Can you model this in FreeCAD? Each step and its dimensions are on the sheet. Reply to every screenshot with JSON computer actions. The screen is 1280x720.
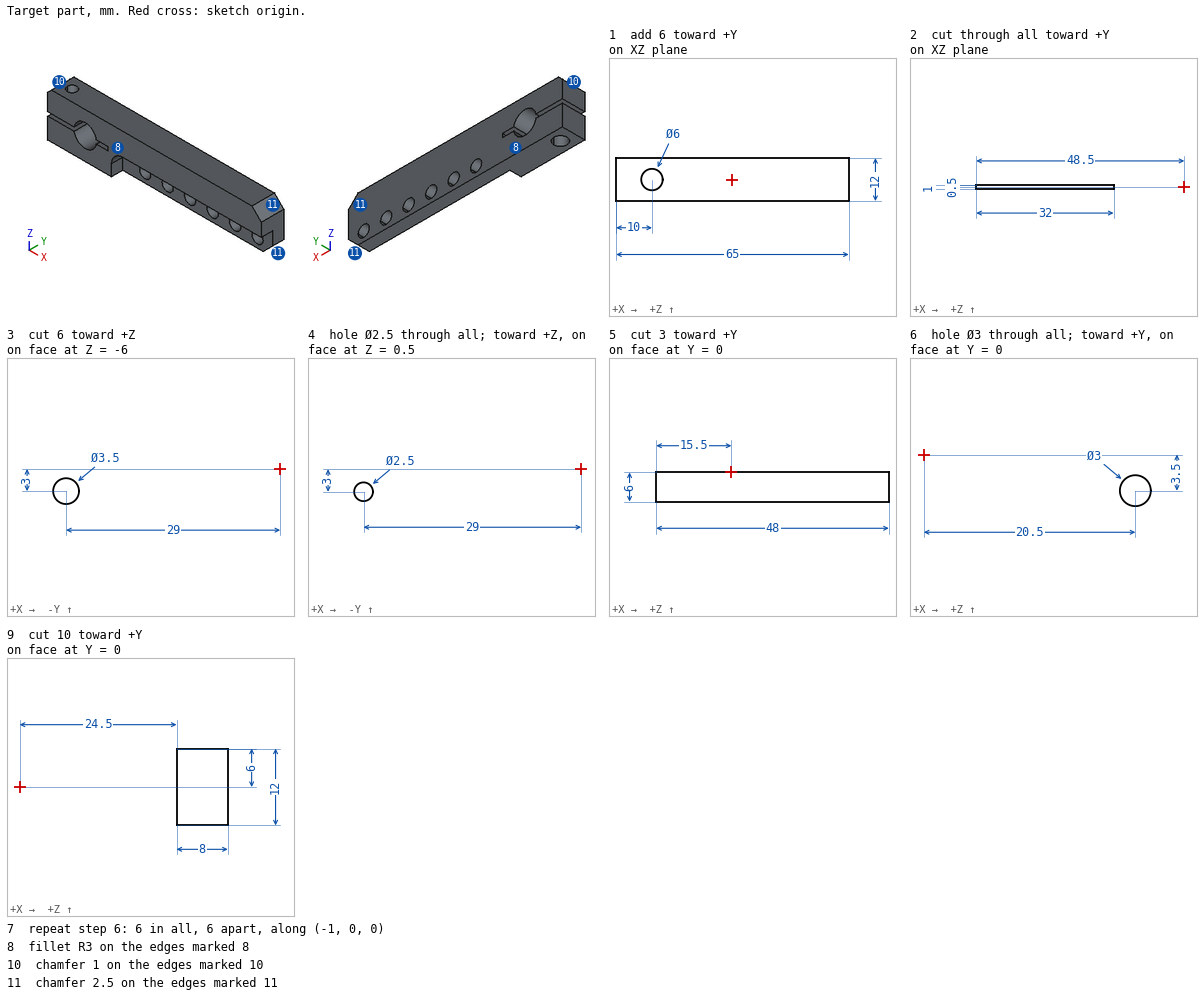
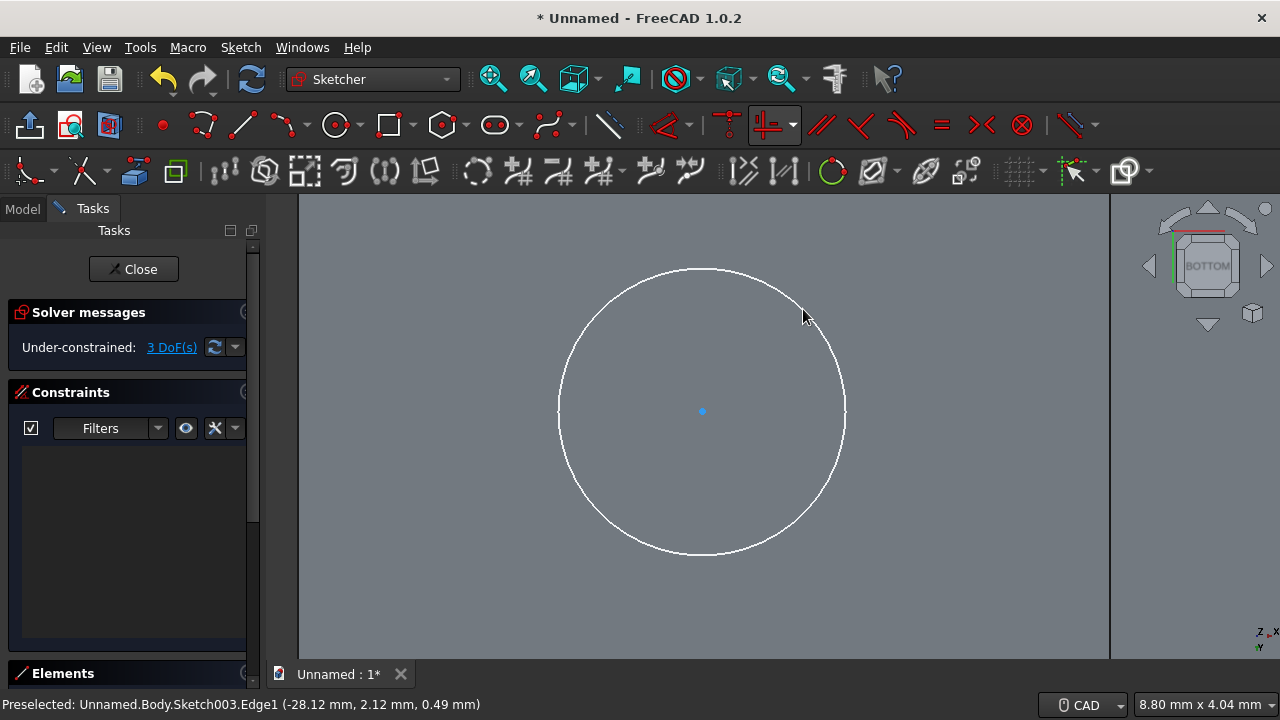
{"action": "left_click", "coordinate": [664, 126]}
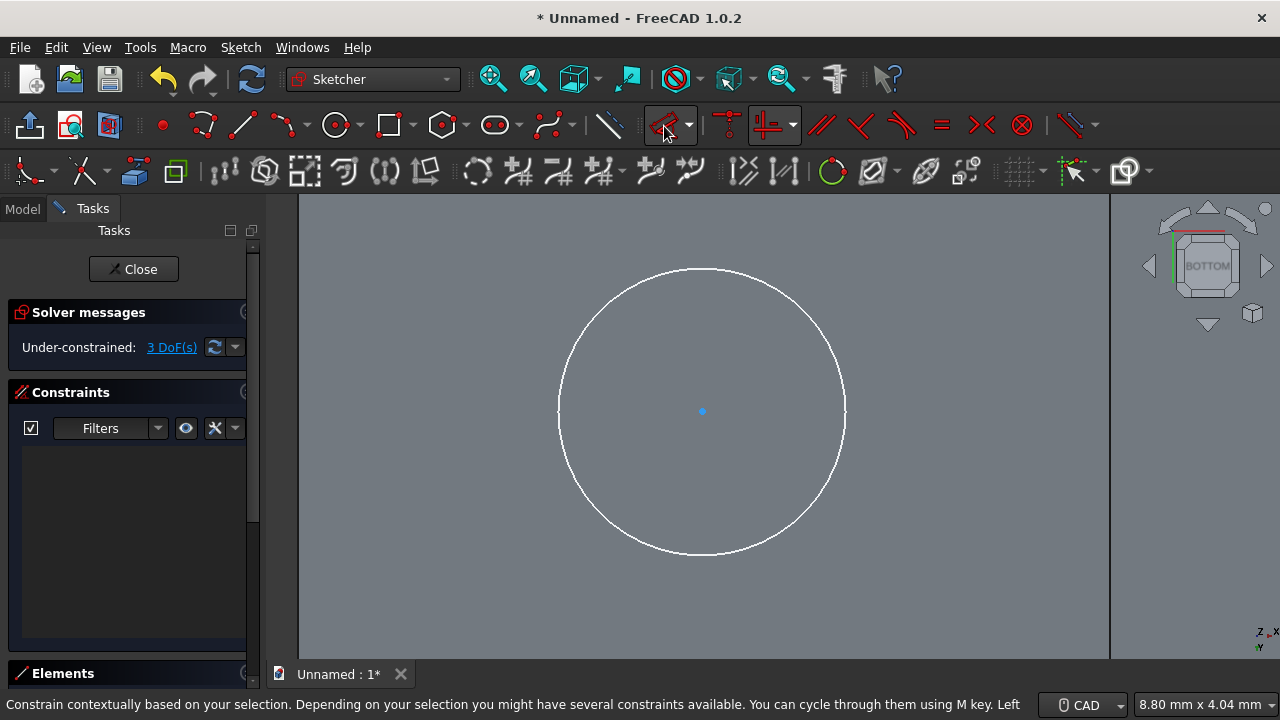
{"action": "left_click", "coordinate": [803, 310]}
{"action": "left_click", "coordinate": [826, 287]}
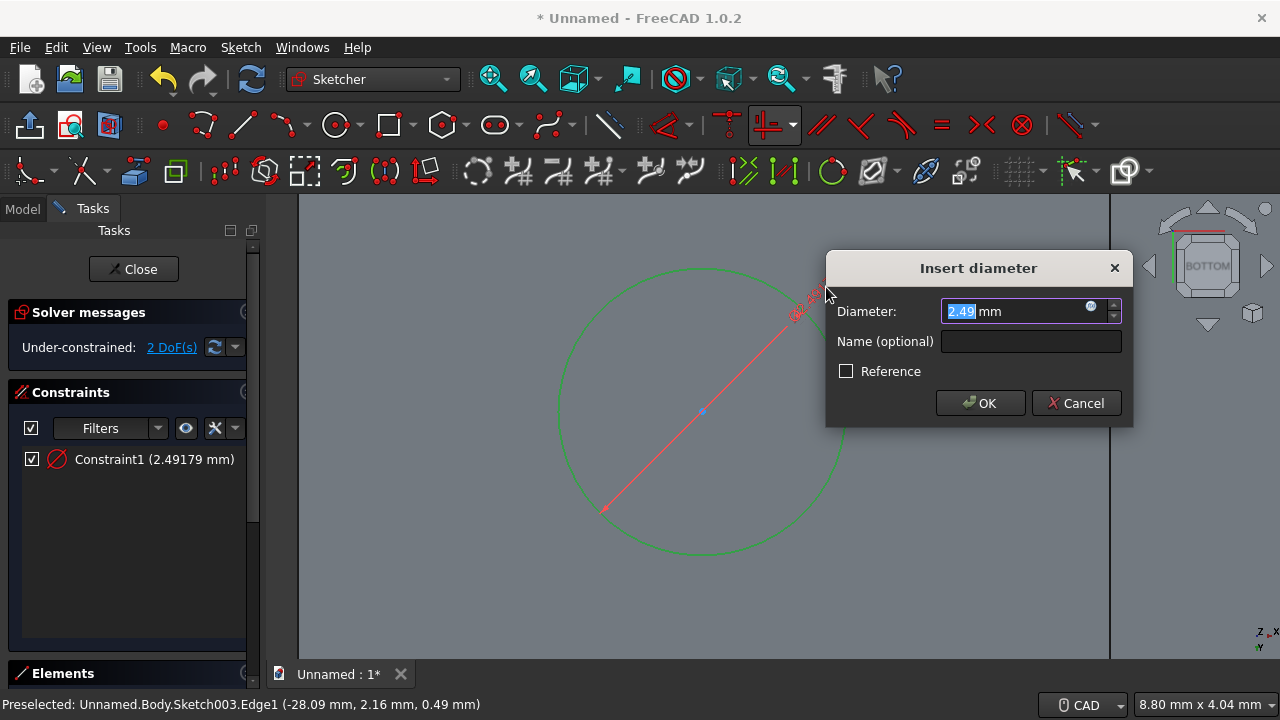
{"action": "type", "text": "2.5"}
{"action": "key", "text": "Return"}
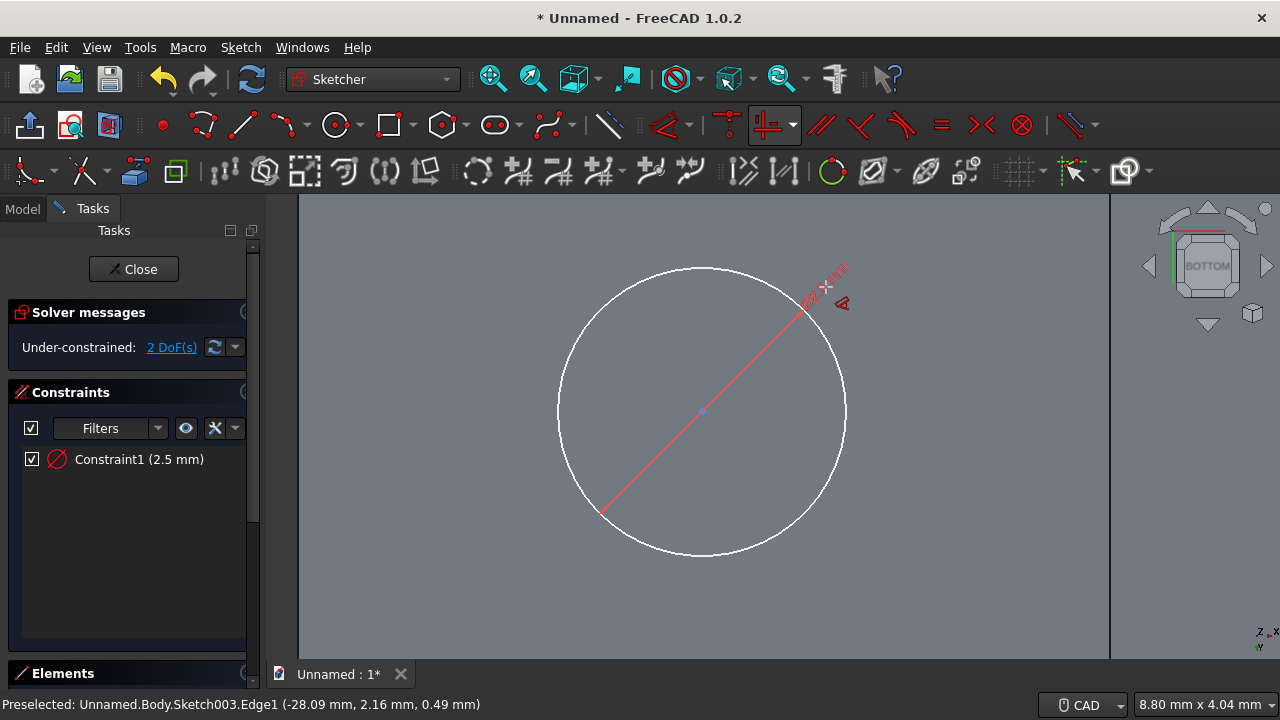
{"action": "left_click", "coordinate": [702, 412]}
{"action": "left_click", "coordinate": [668, 317]}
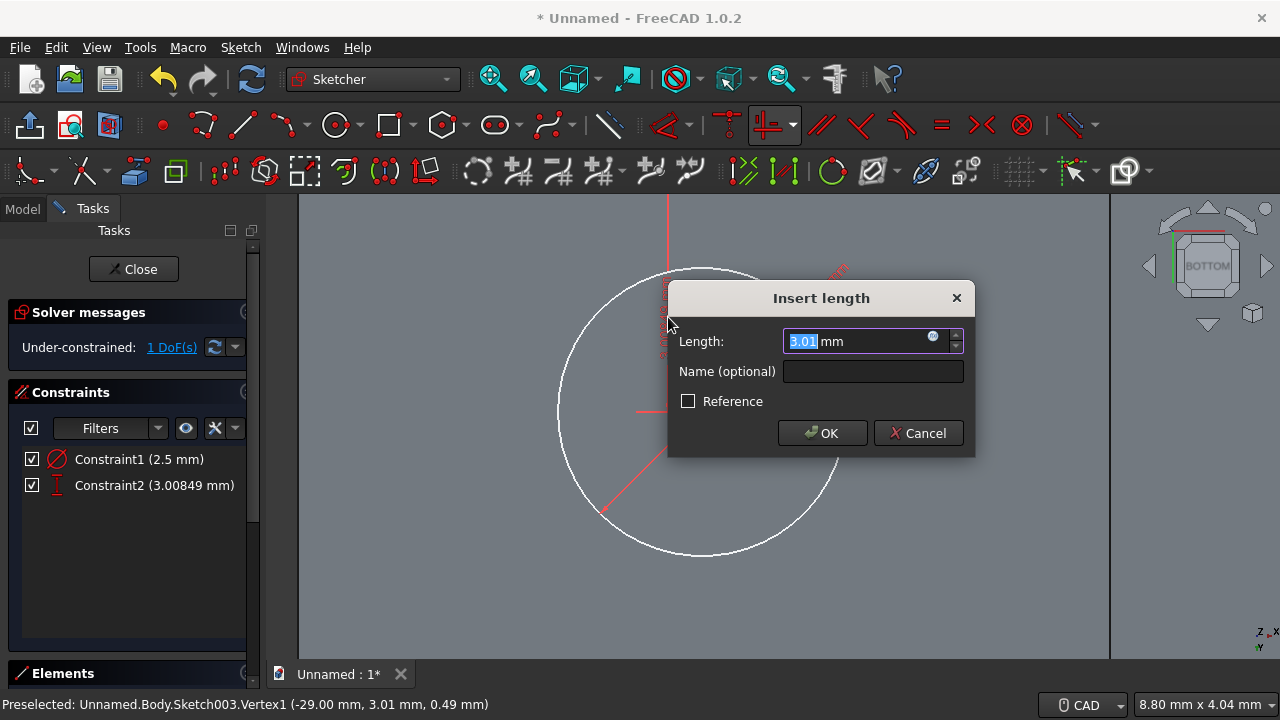
{"action": "type", "text": "3"}
{"action": "key", "text": "Return"}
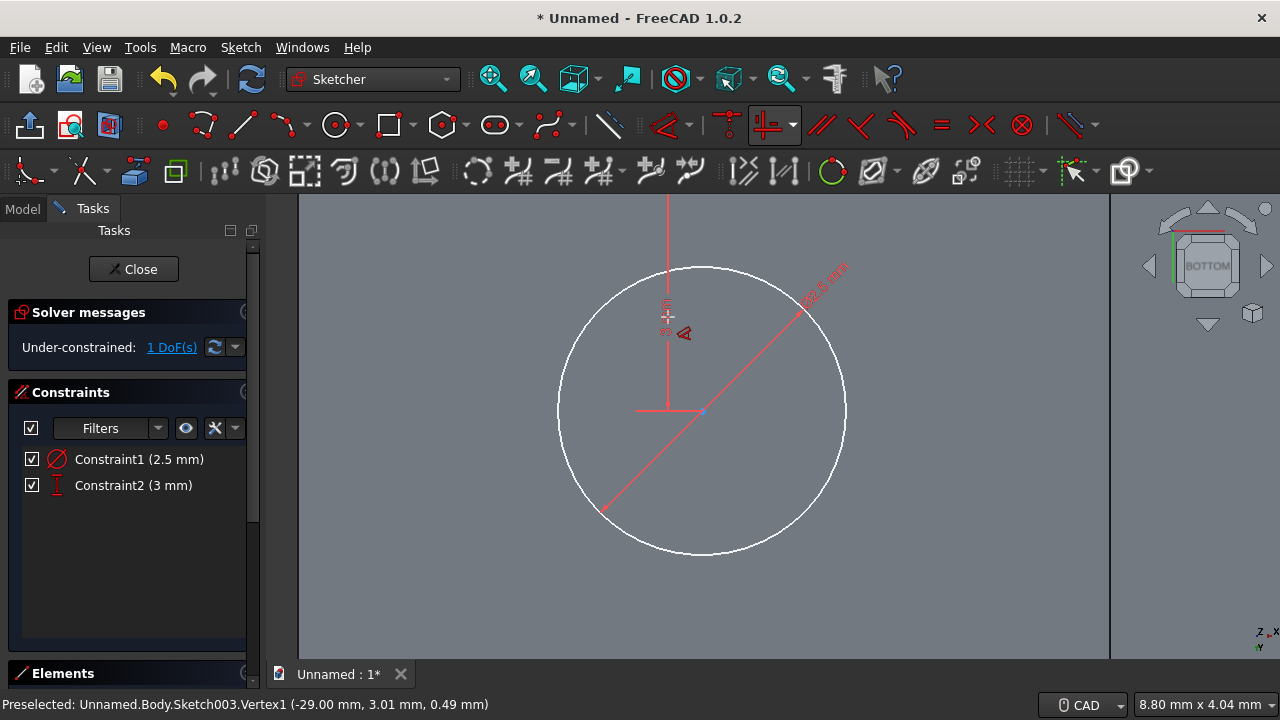
{"action": "left_click", "coordinate": [702, 411]}
{"action": "left_click", "coordinate": [909, 445]}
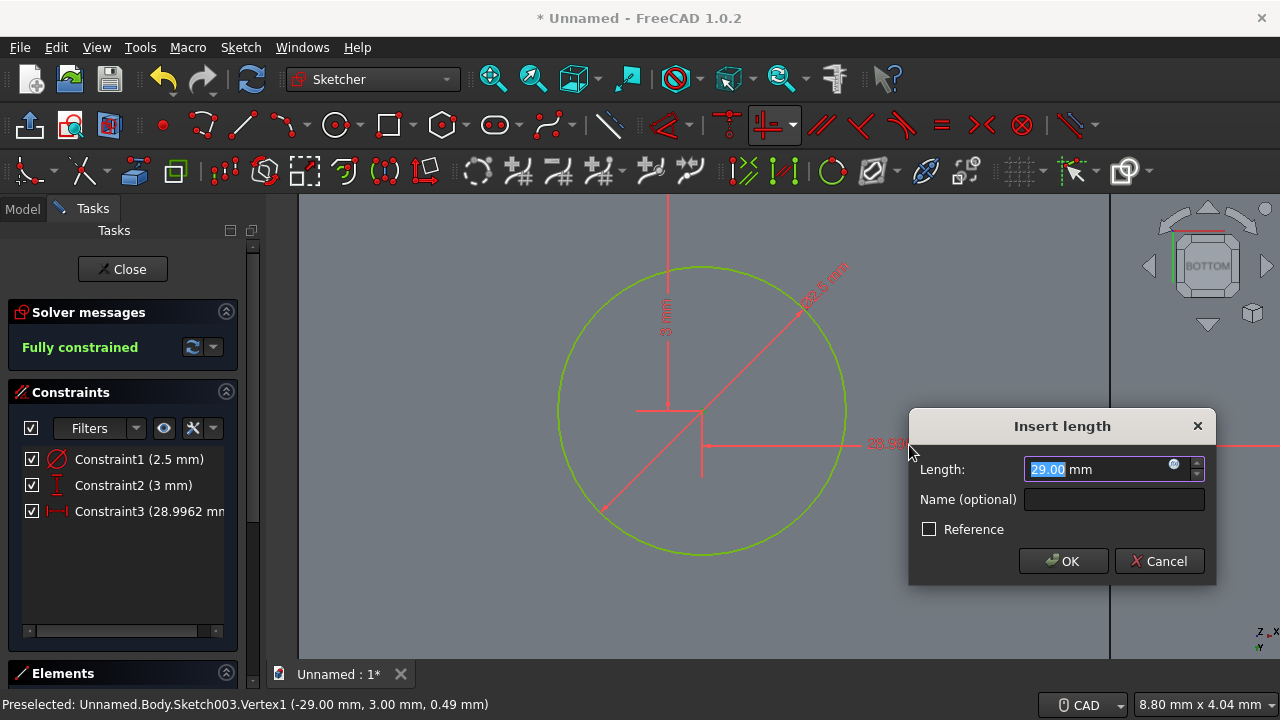
{"action": "type", "text": "29"}
{"action": "key", "text": "Return"}
{"action": "key", "text": "Escape"}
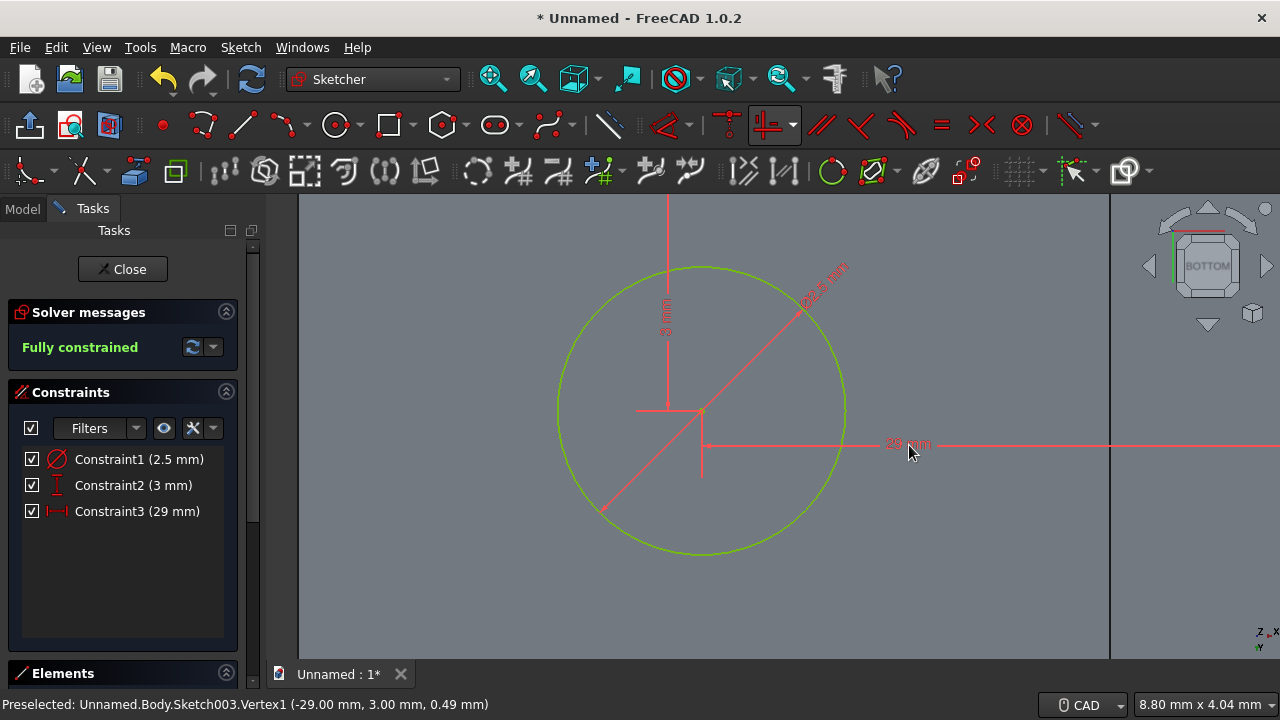
{"action": "left_click", "coordinate": [123, 269]}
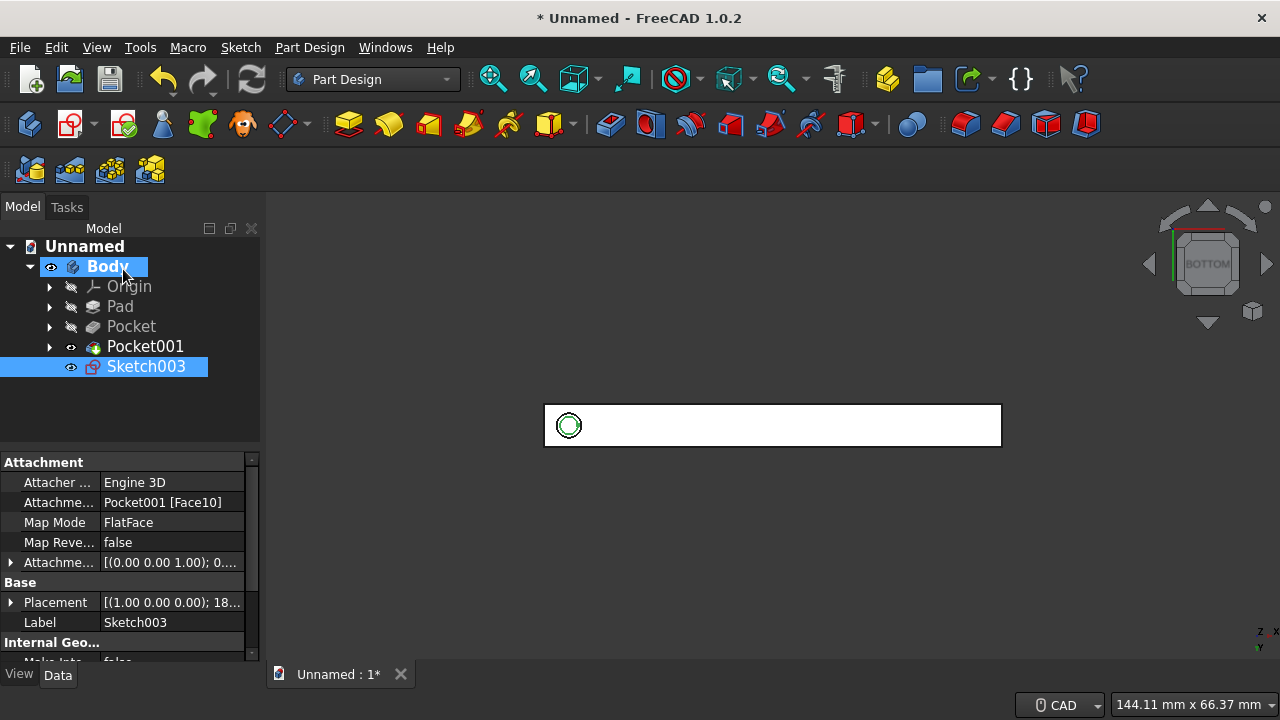
{"action": "left_click", "coordinate": [652, 124]}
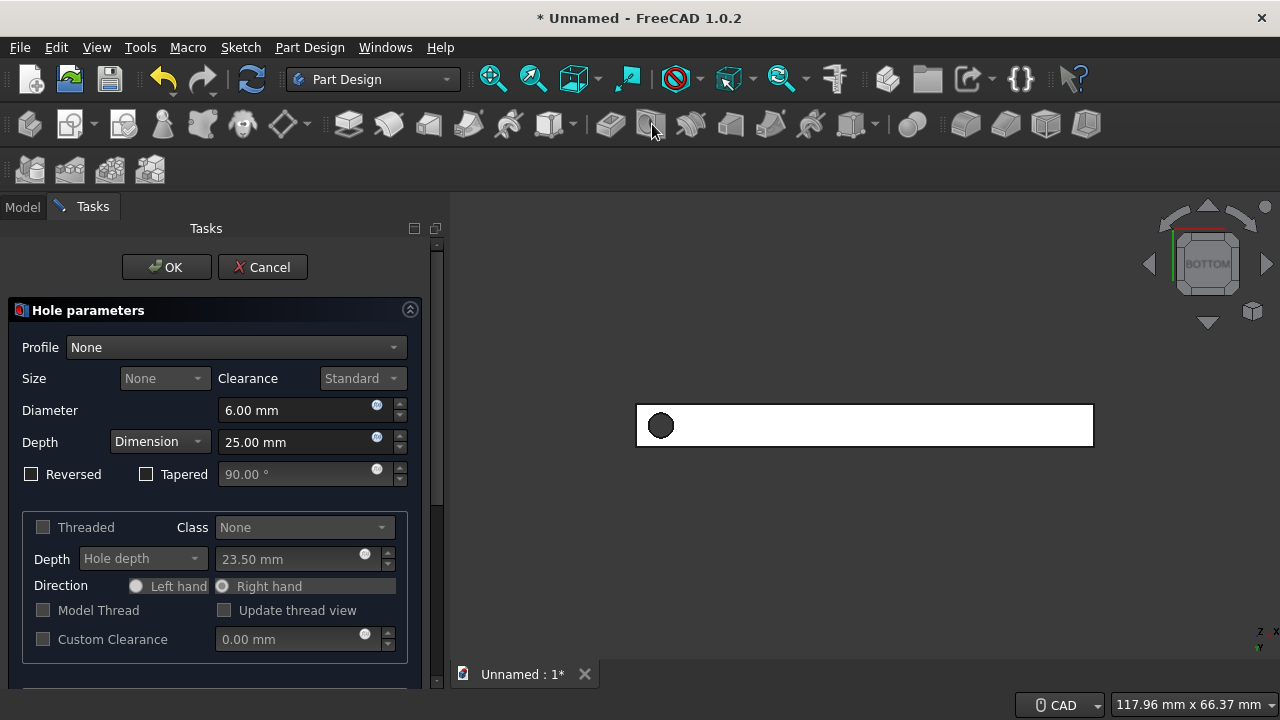
{"action": "triple_click", "coordinate": [305, 410]}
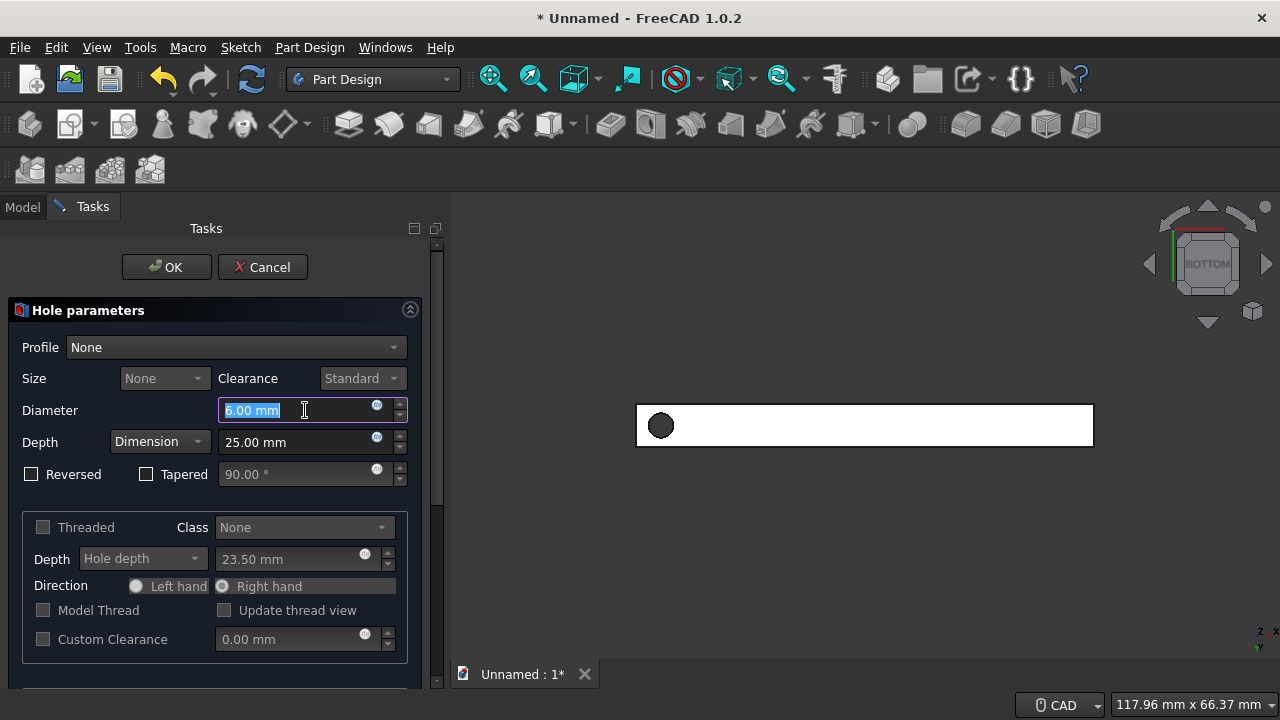
{"action": "type", "text": "2.5"}
{"action": "key", "text": "Tab"}